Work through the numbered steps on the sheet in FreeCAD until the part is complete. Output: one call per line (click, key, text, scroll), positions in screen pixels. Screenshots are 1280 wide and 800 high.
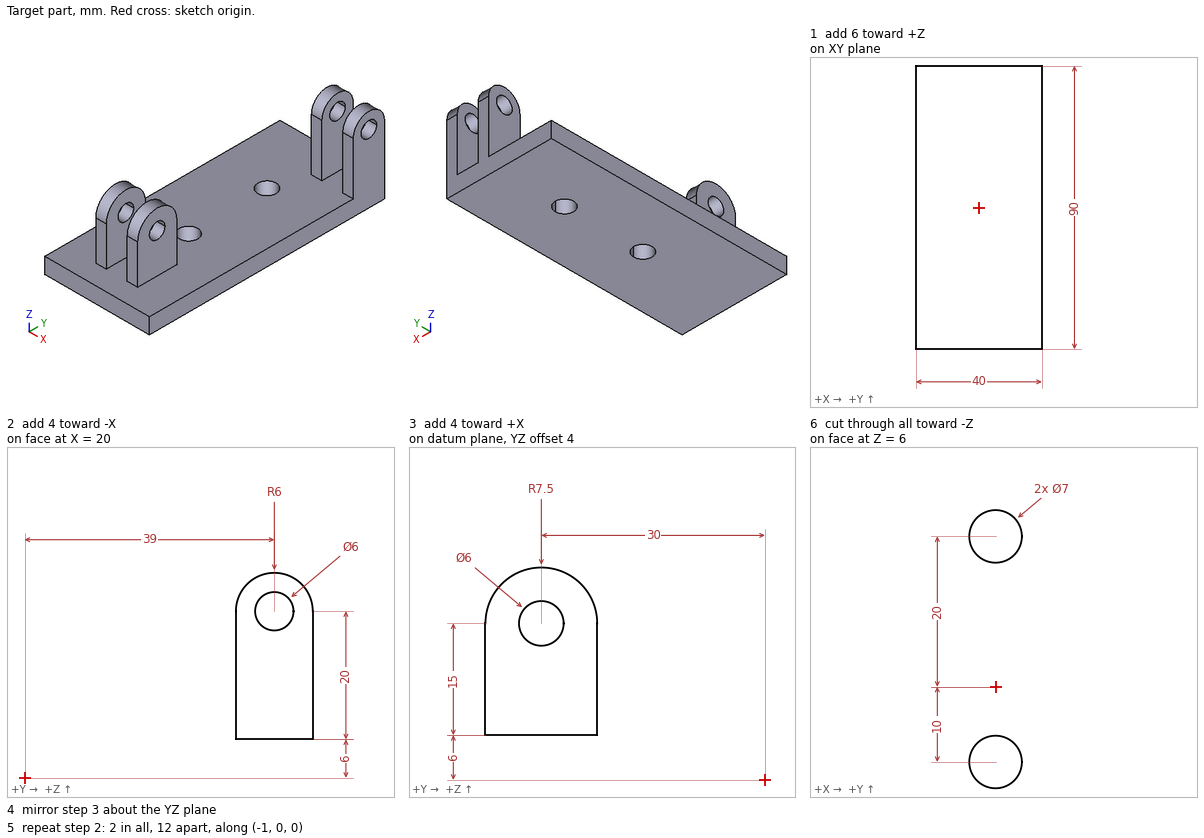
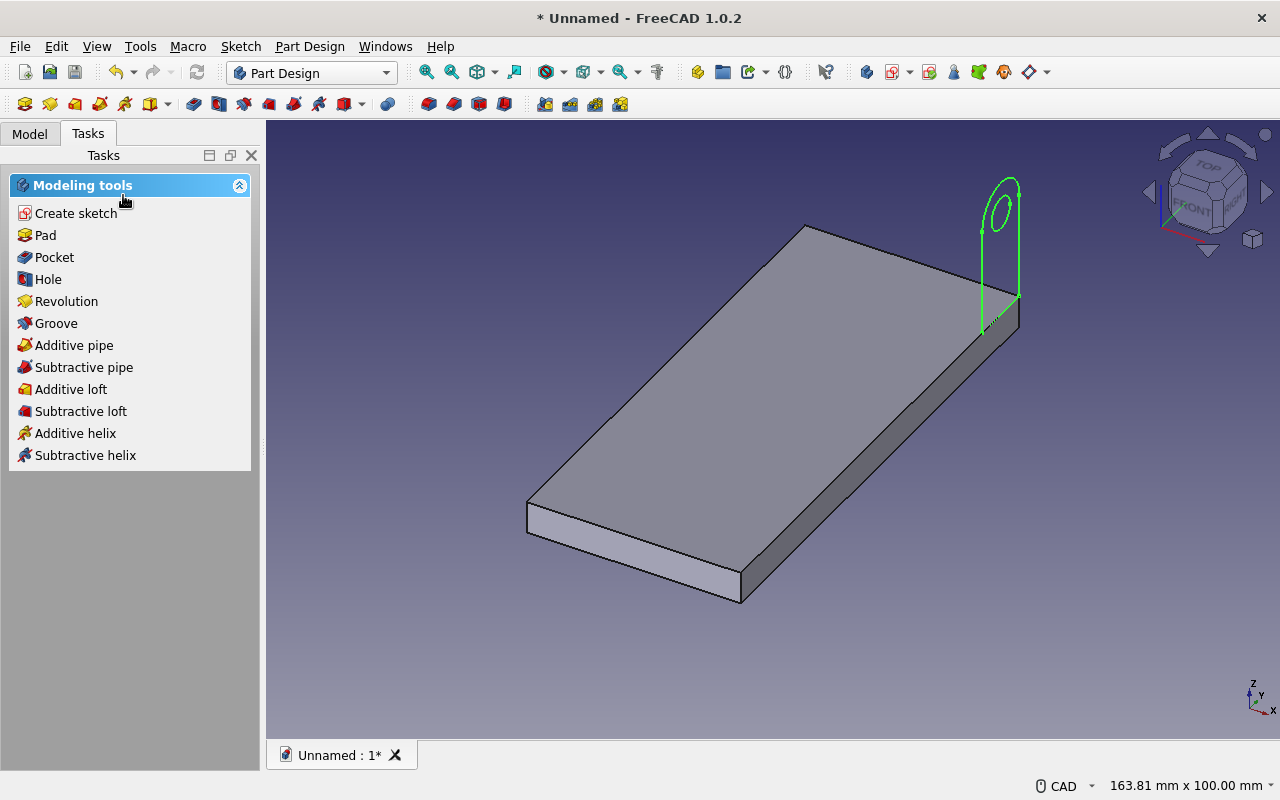
click(25, 104)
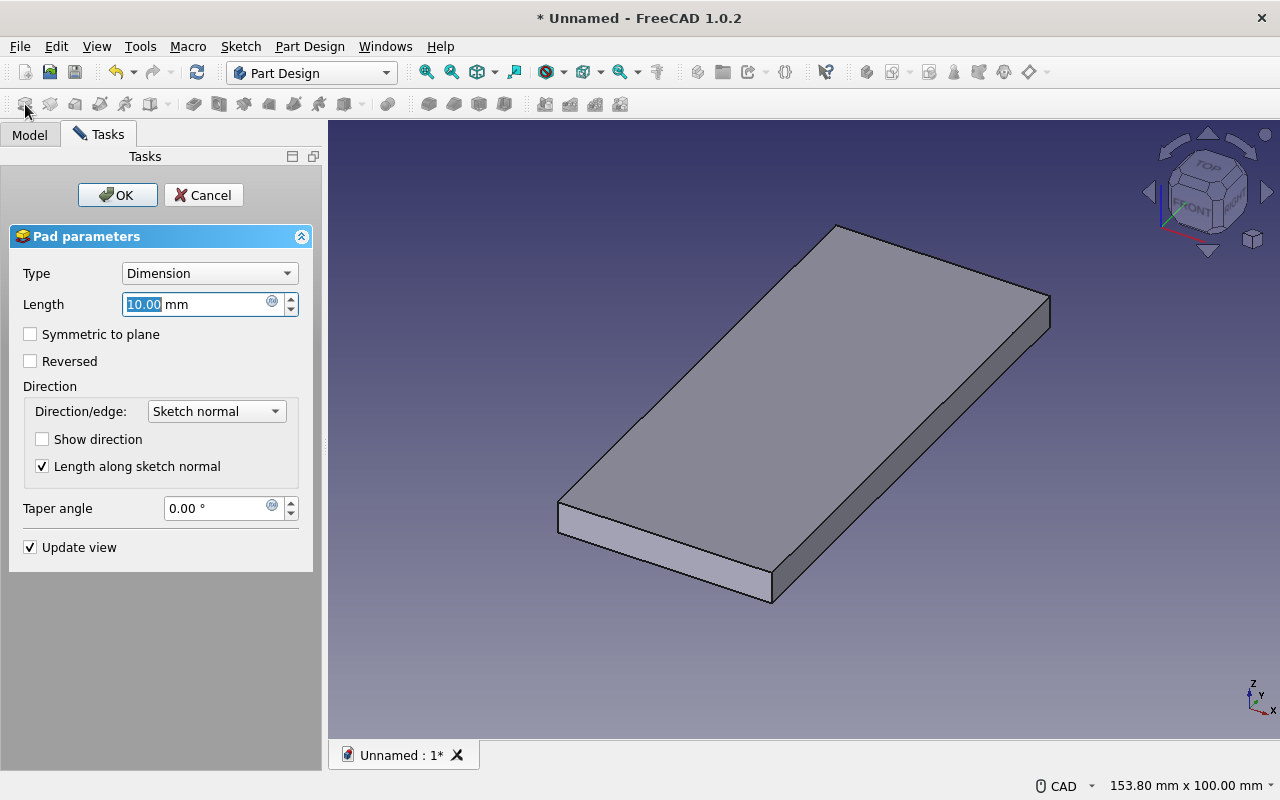
text(4)
key(Tab)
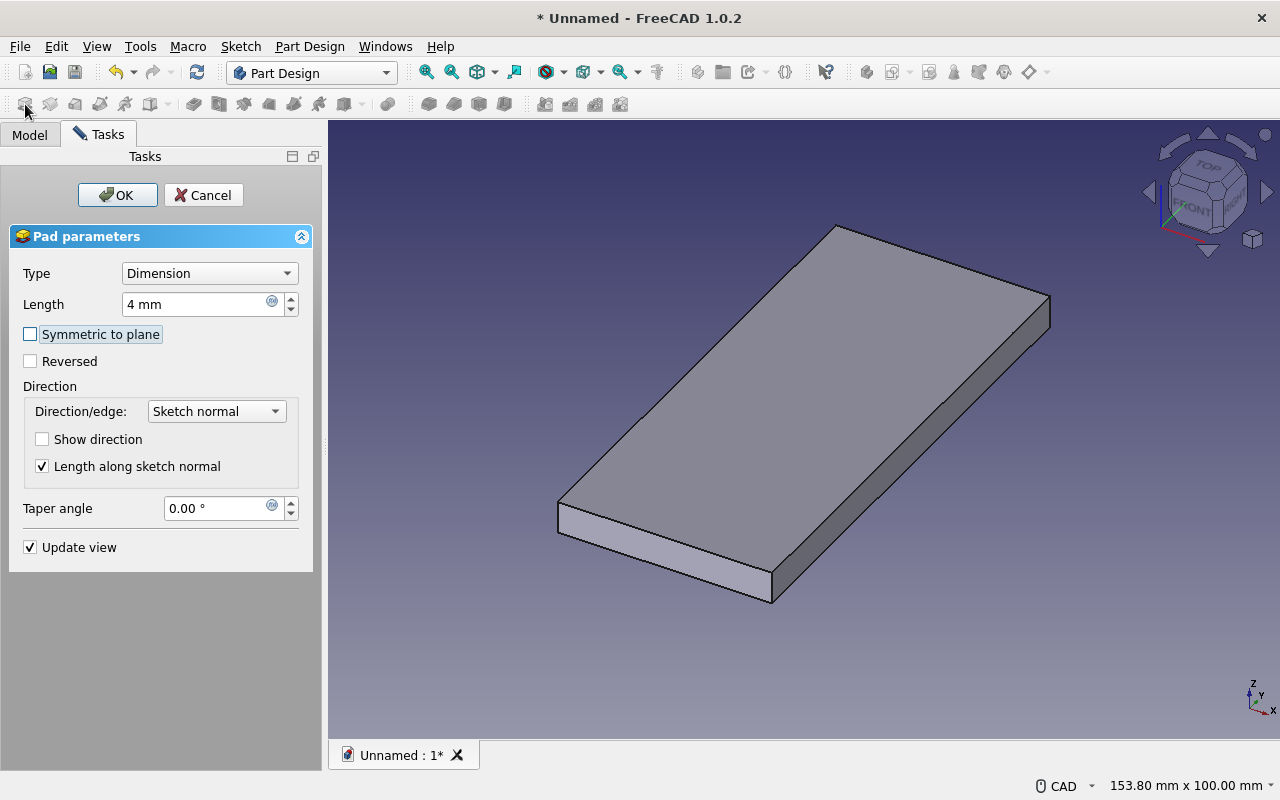
click(31, 361)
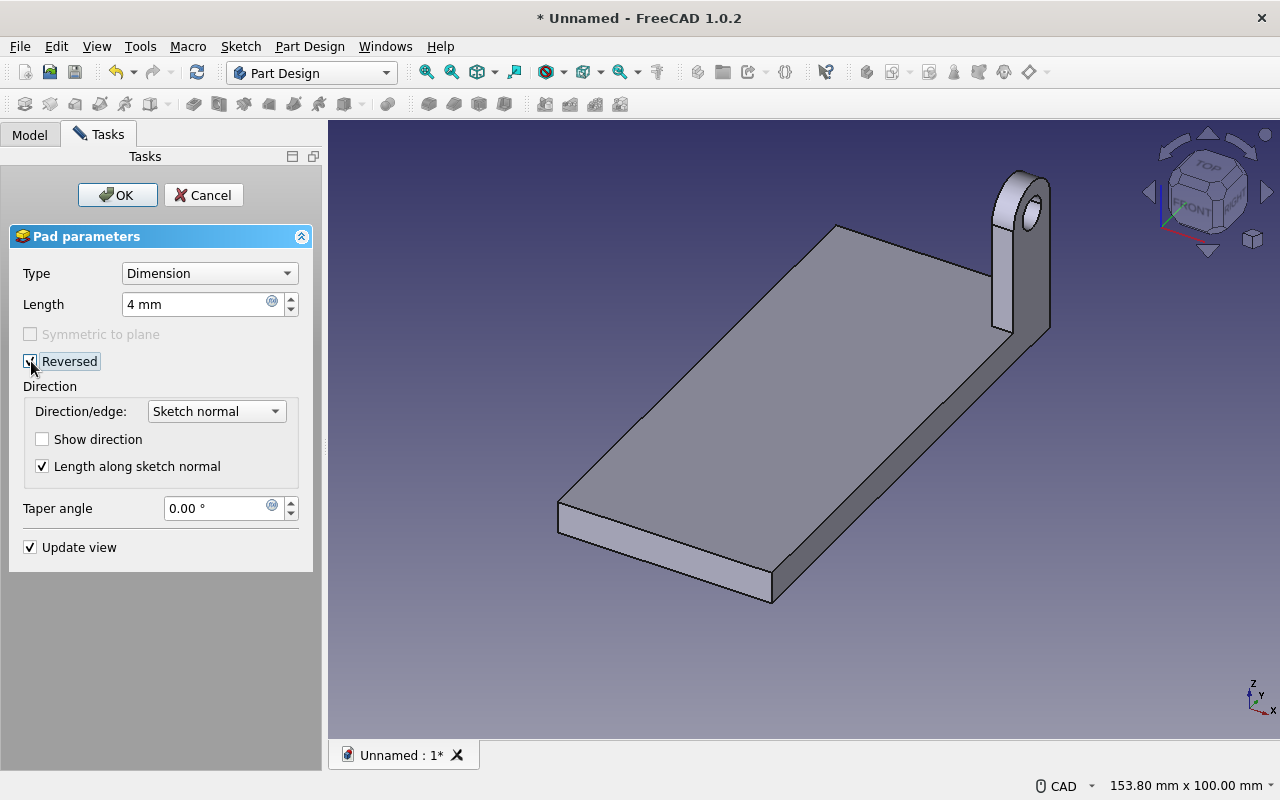
click(118, 195)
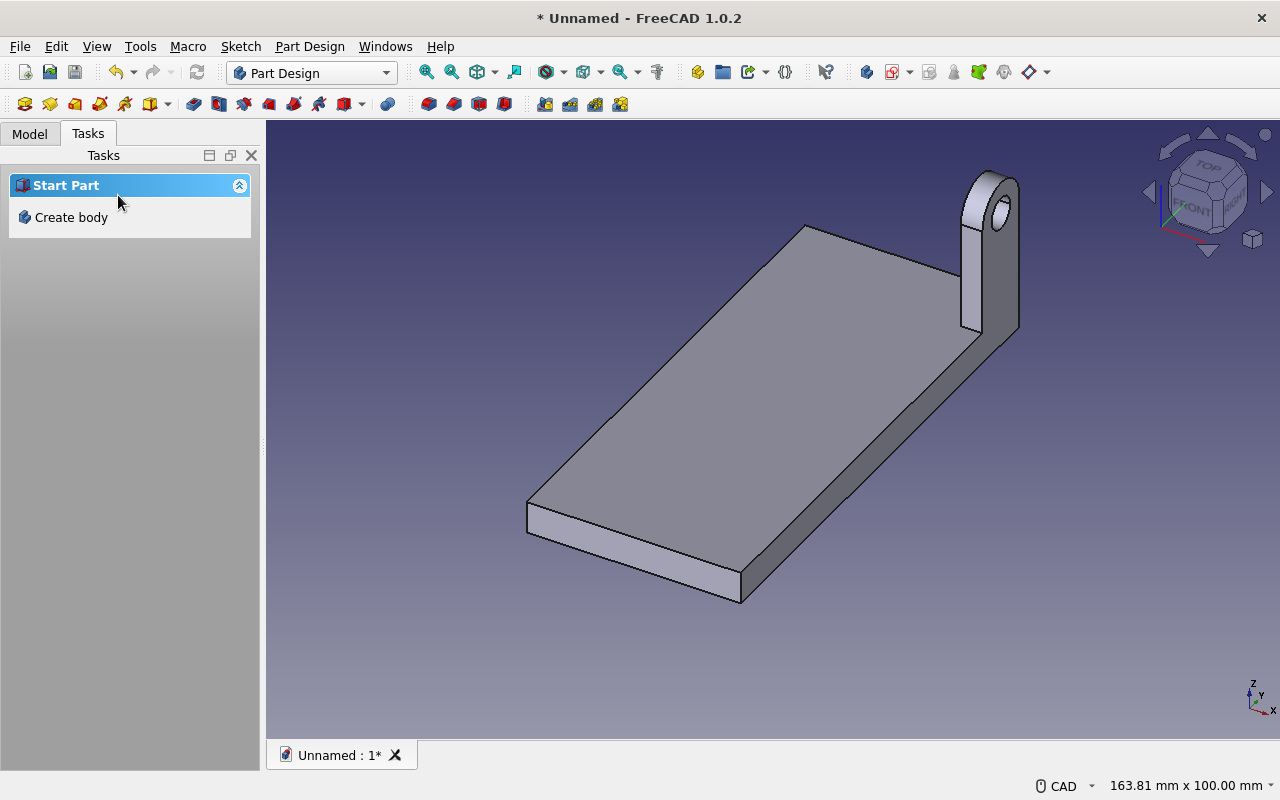
click(427, 72)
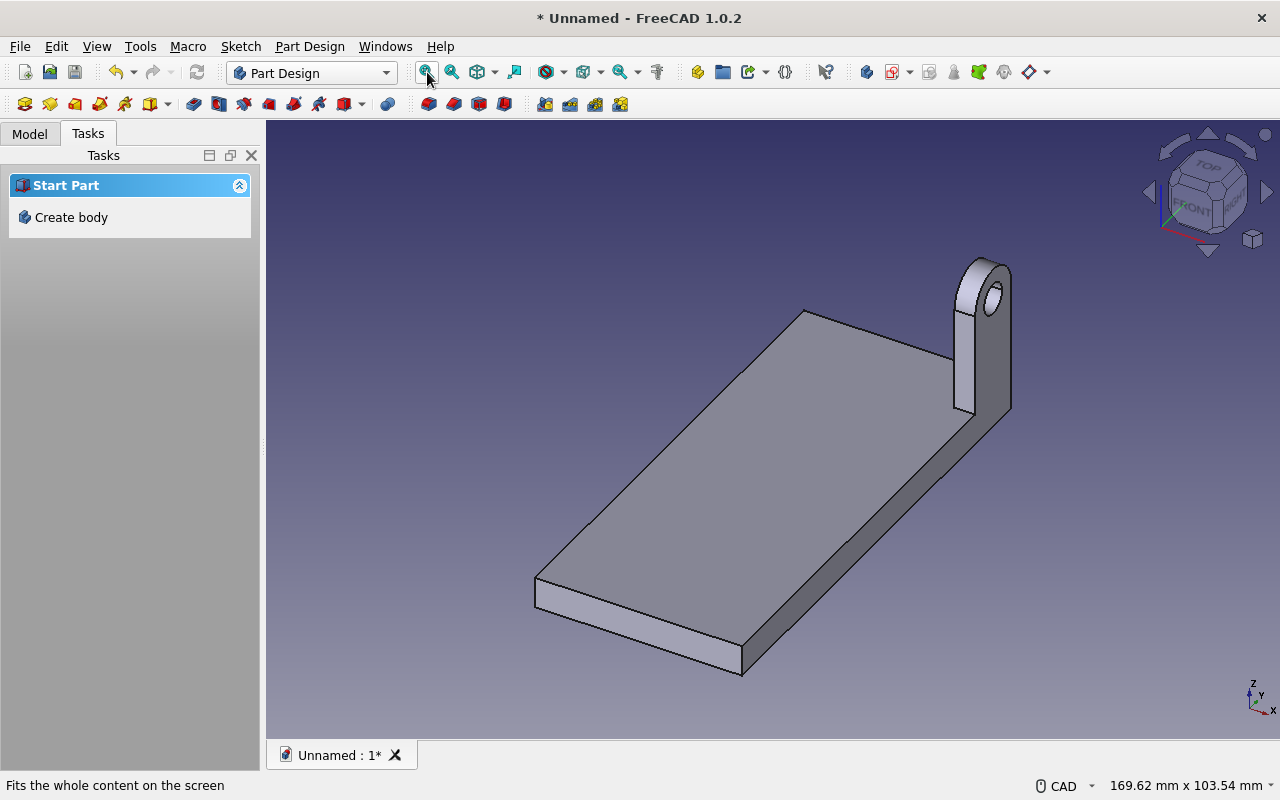
click(30, 134)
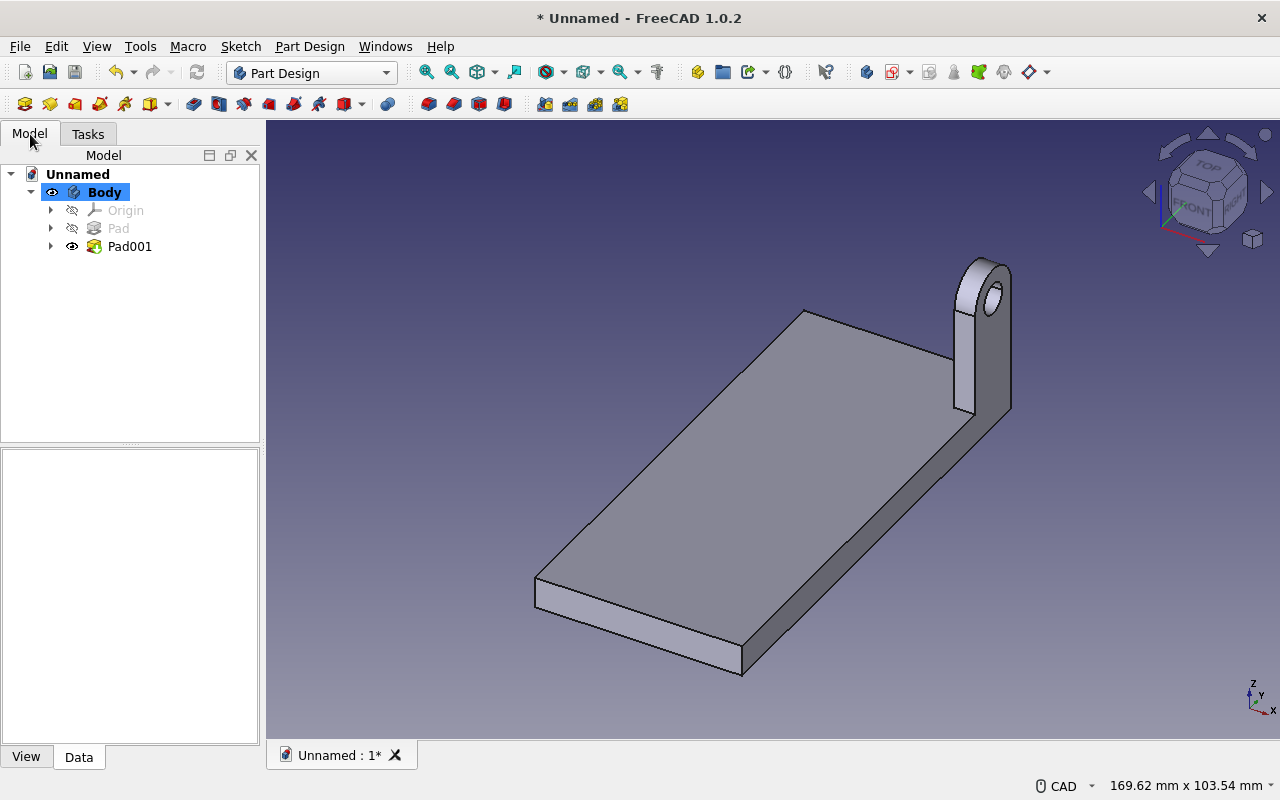
click(51, 210)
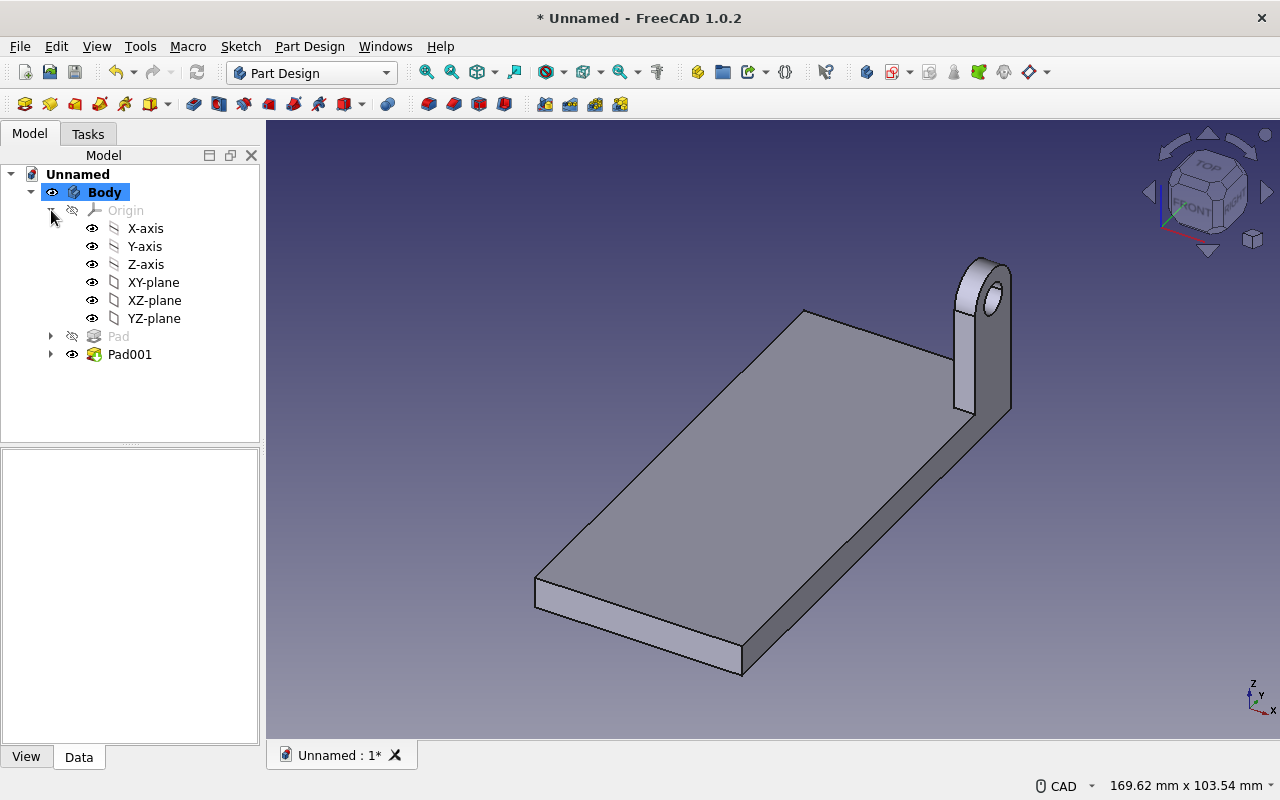
click(137, 318)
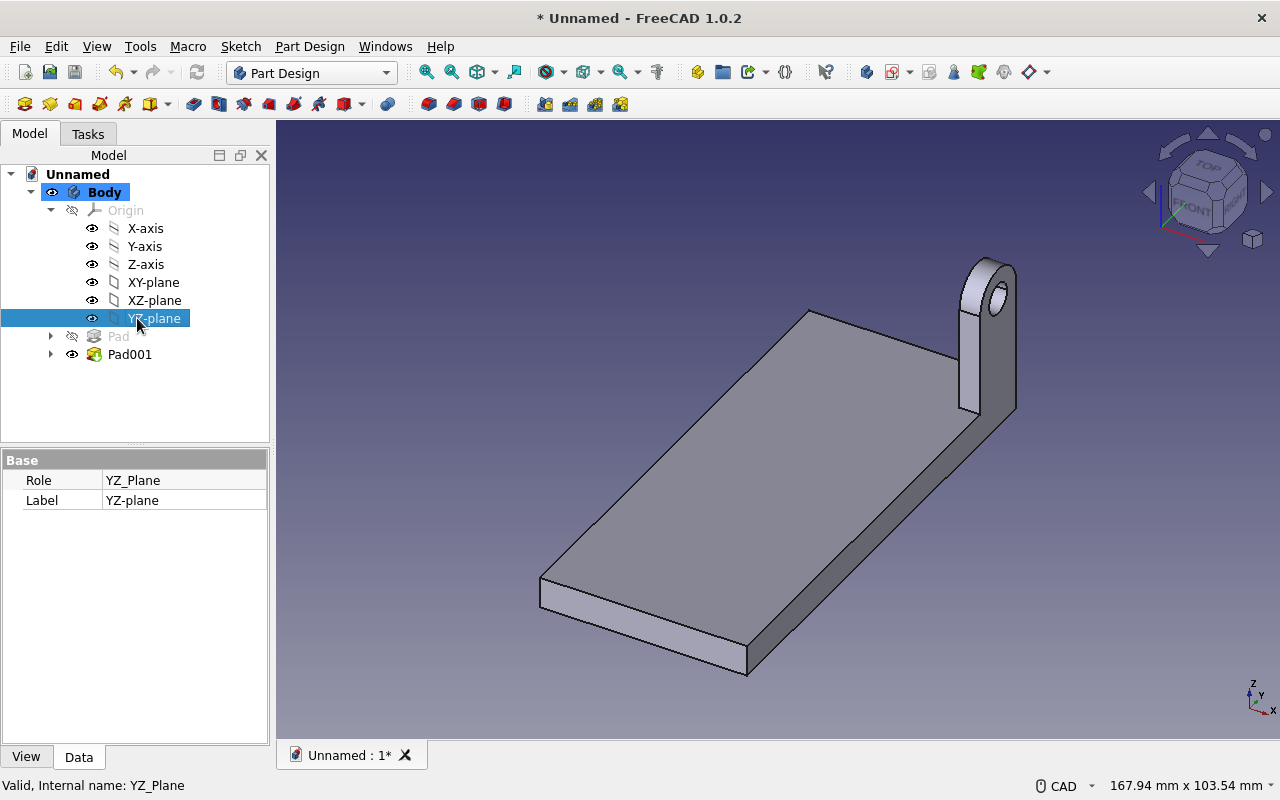
click(1028, 72)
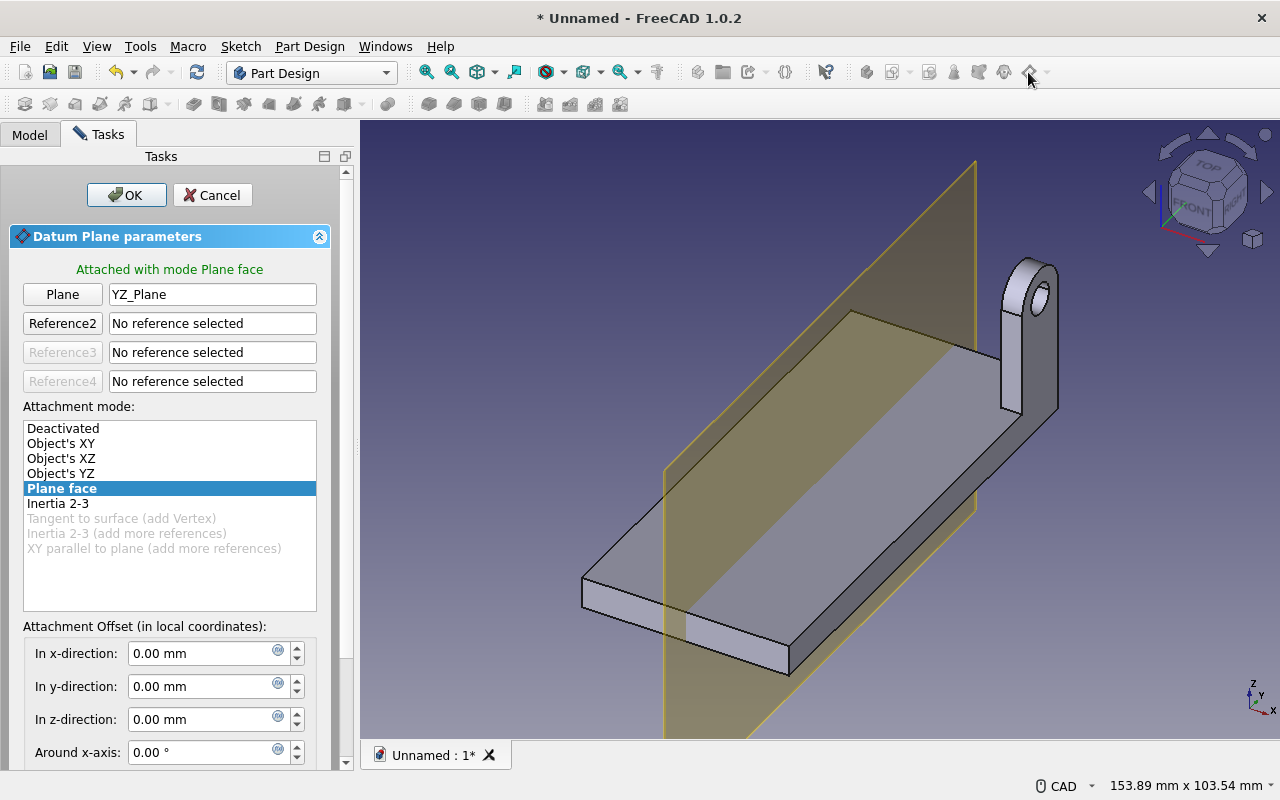
triple_click(210, 720)